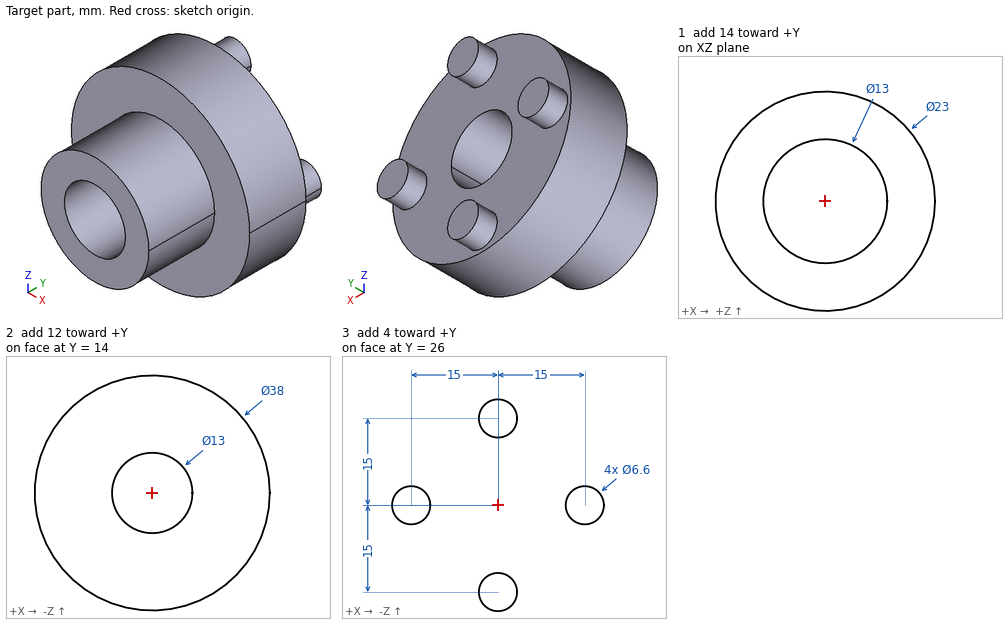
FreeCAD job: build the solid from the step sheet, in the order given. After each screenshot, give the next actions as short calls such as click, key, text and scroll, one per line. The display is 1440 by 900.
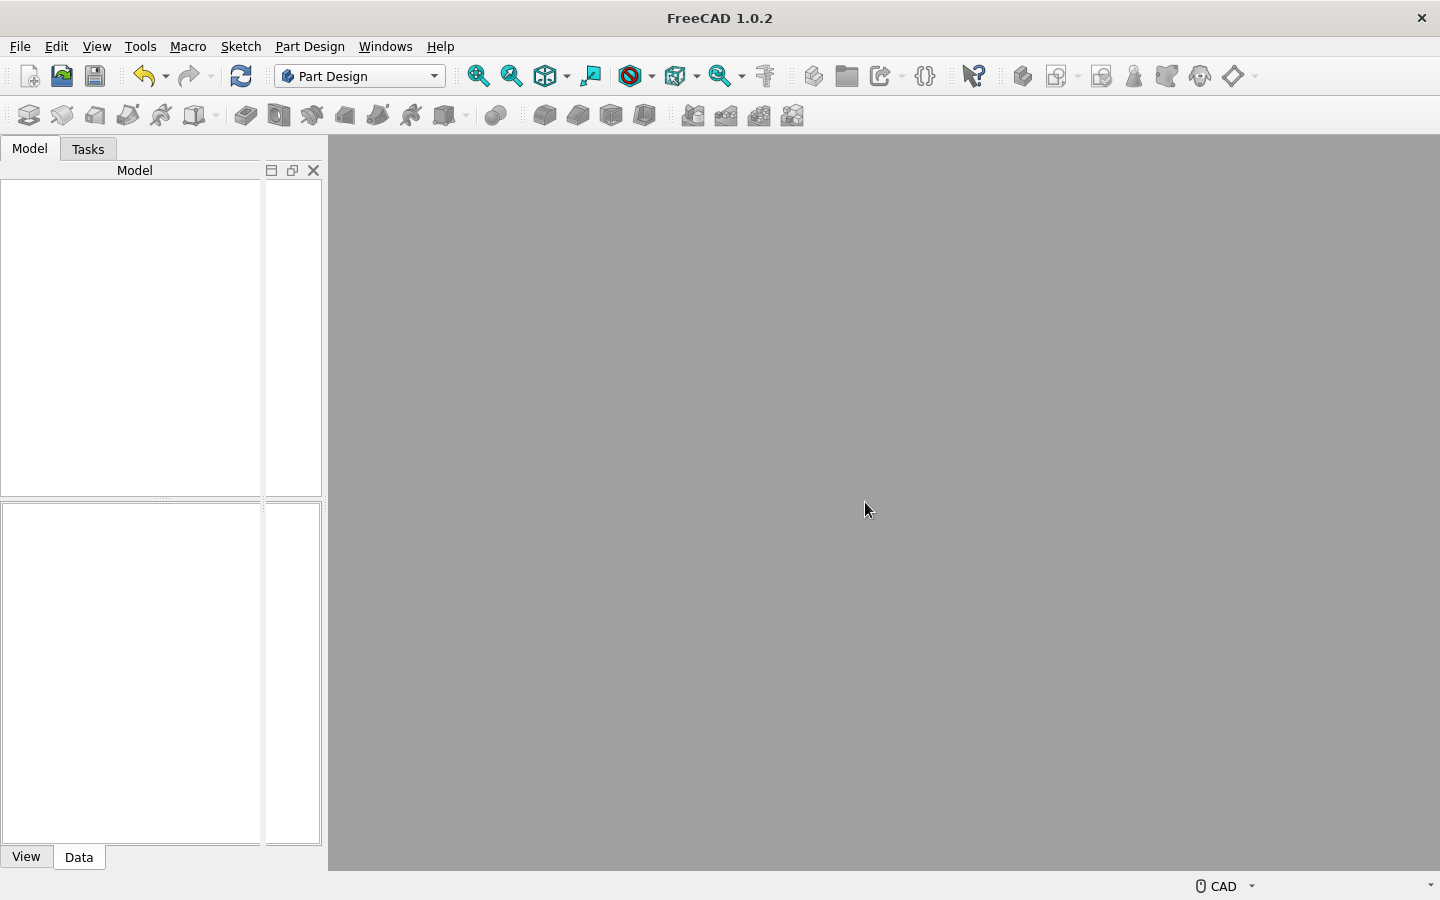
click(29, 76)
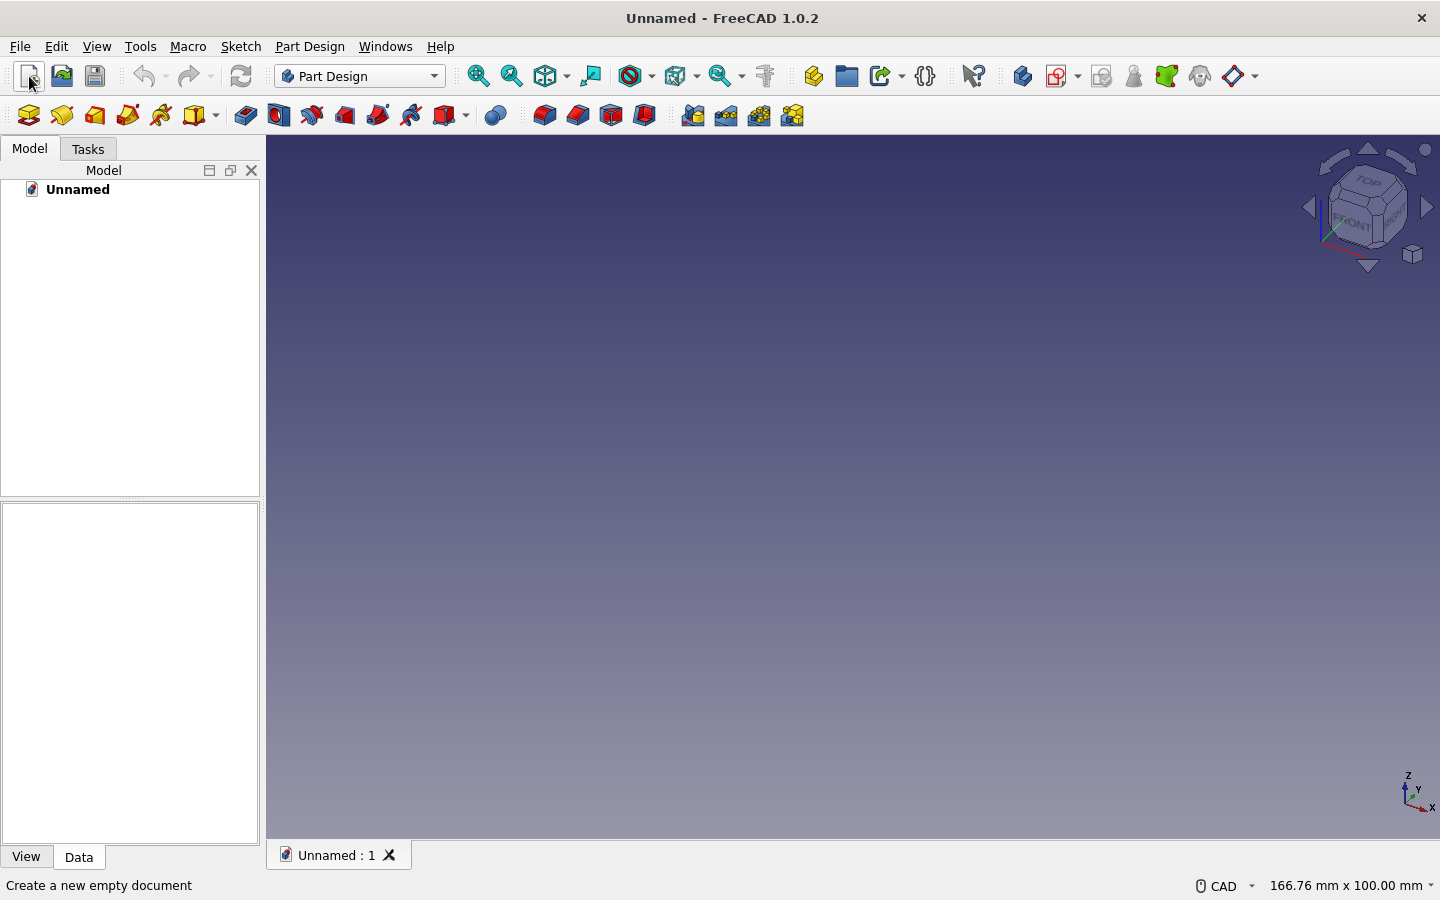
click(1056, 76)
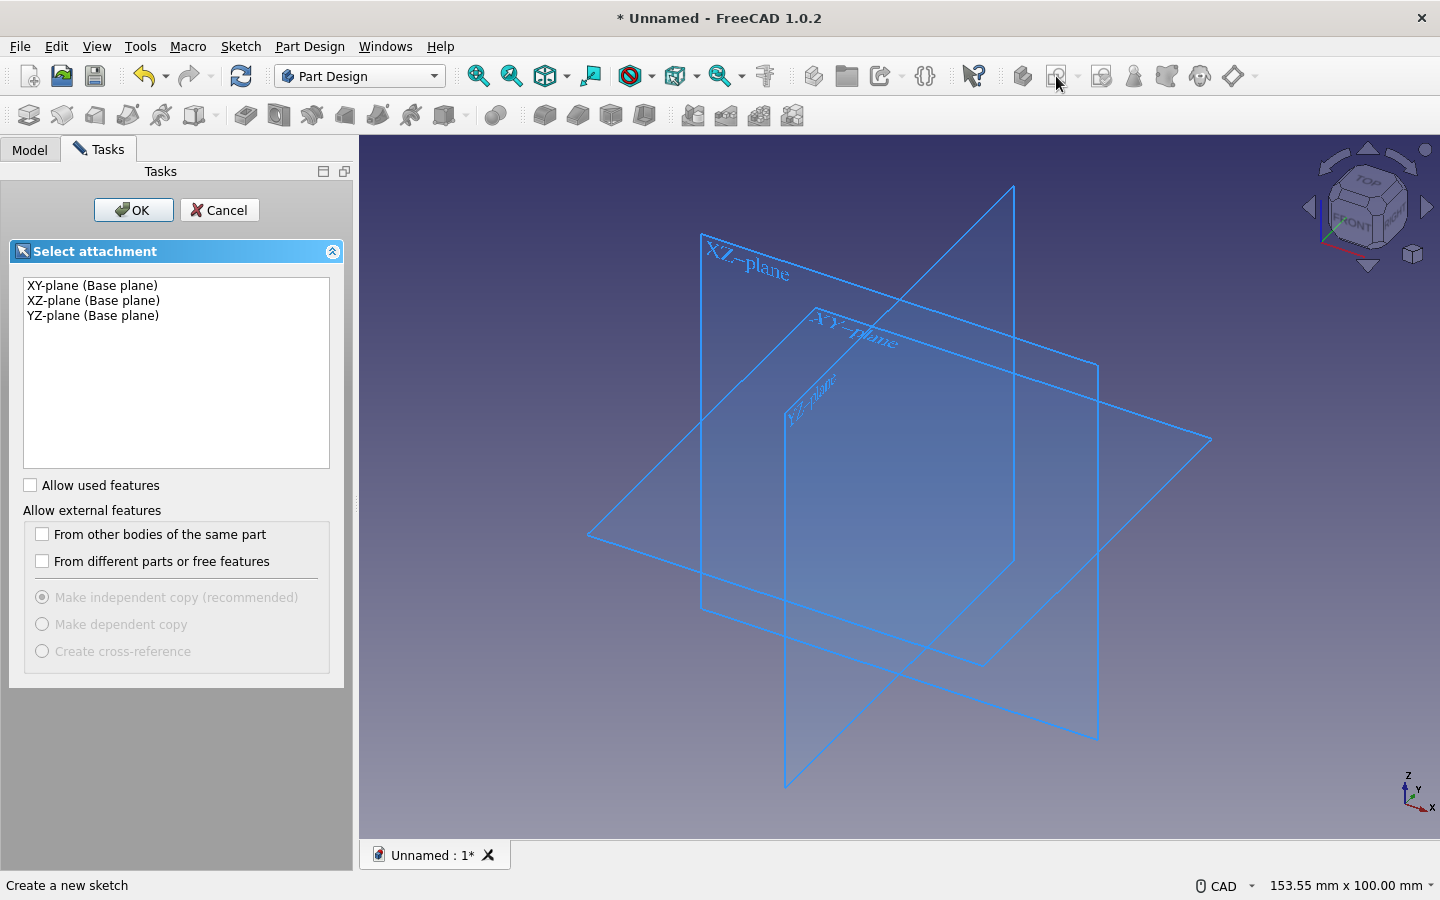
click(84, 300)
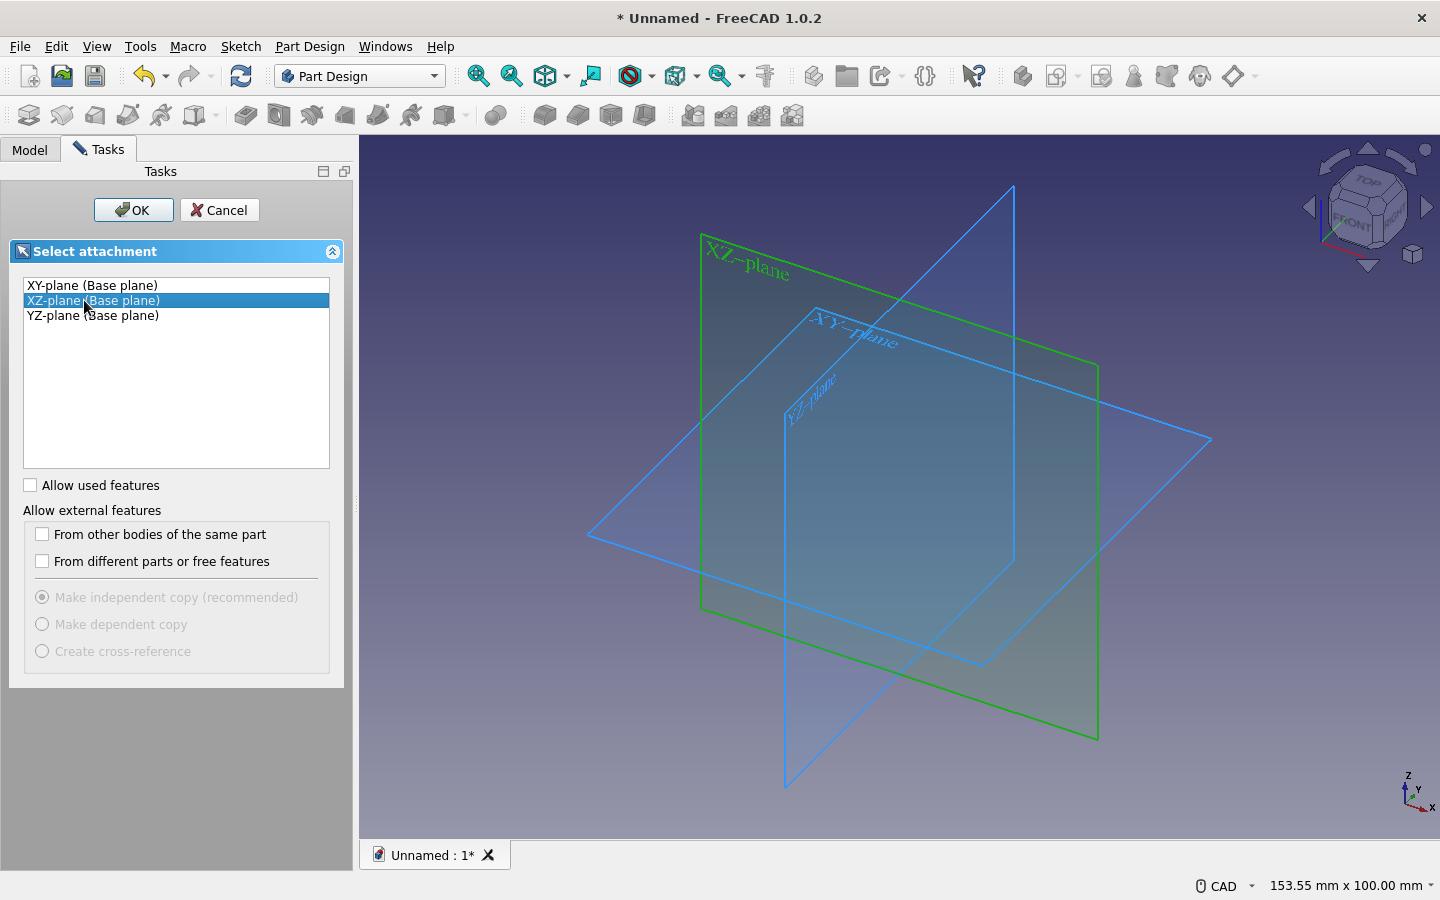
click(134, 210)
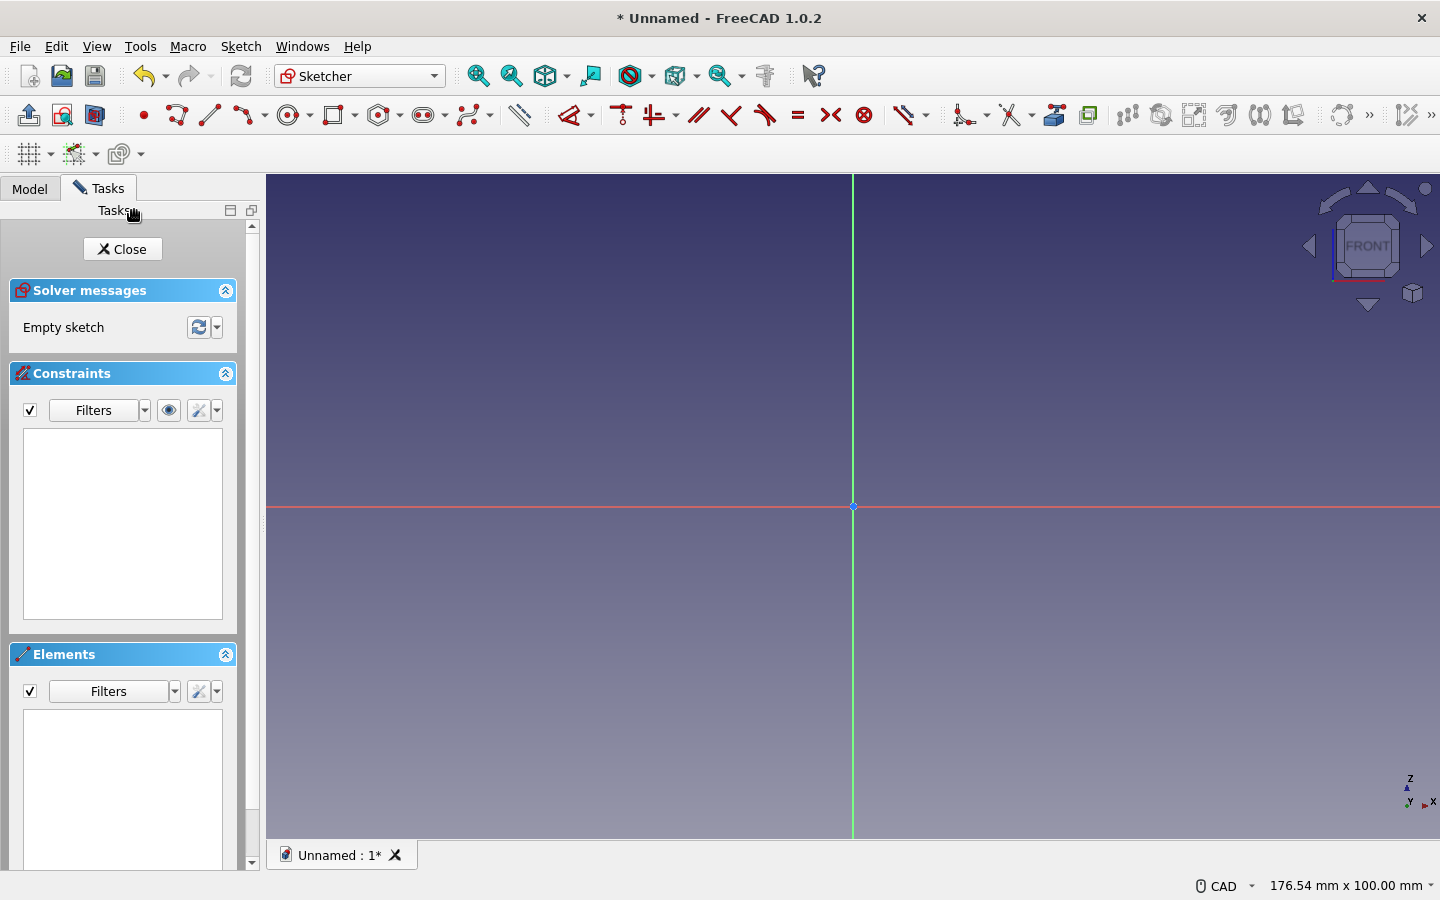
scroll(893, 507, up, 5)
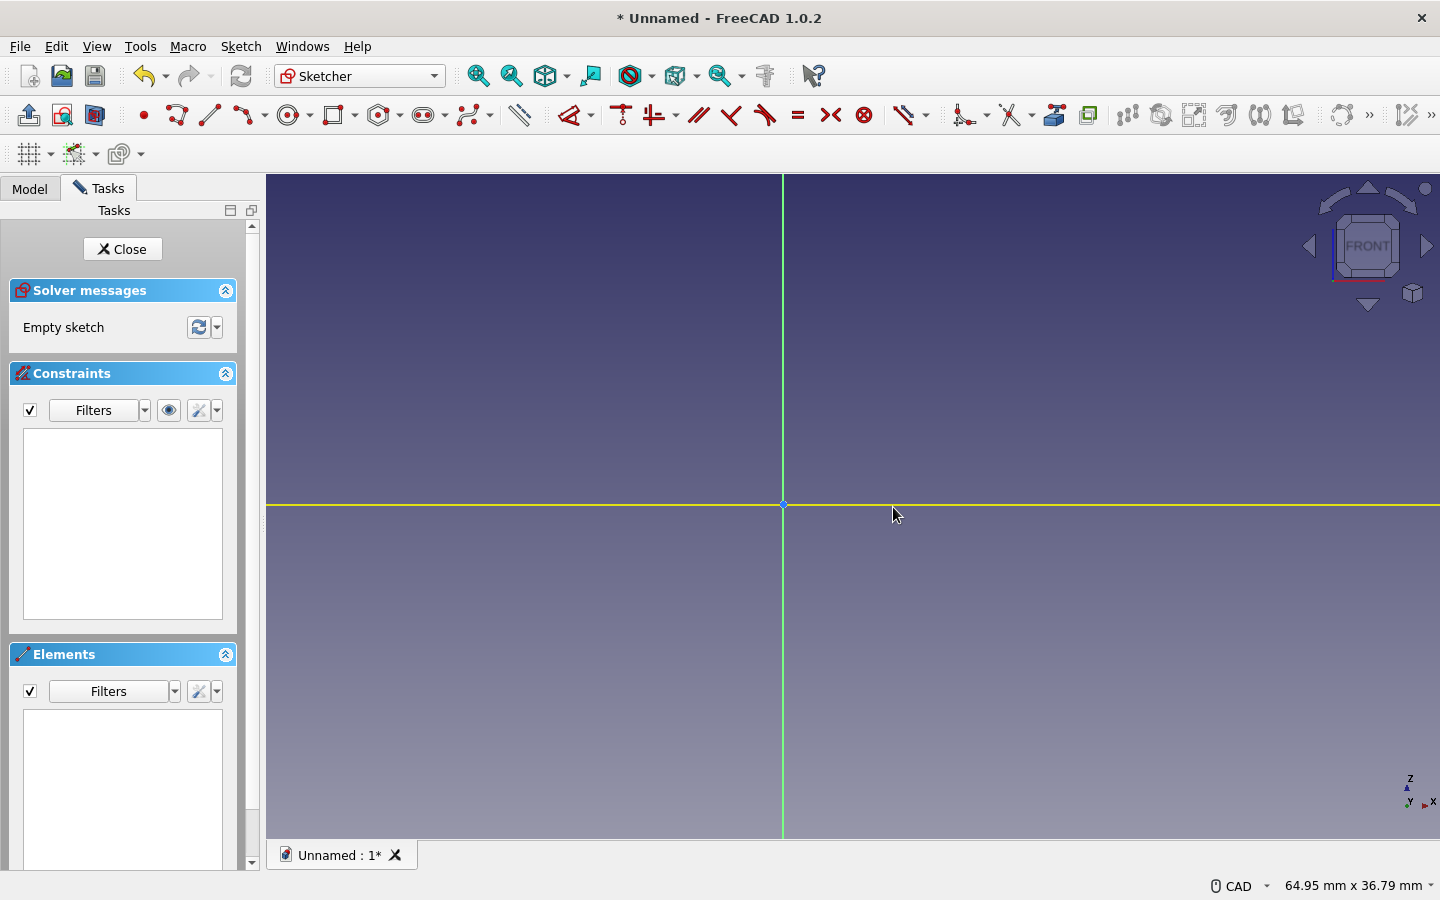
click(288, 116)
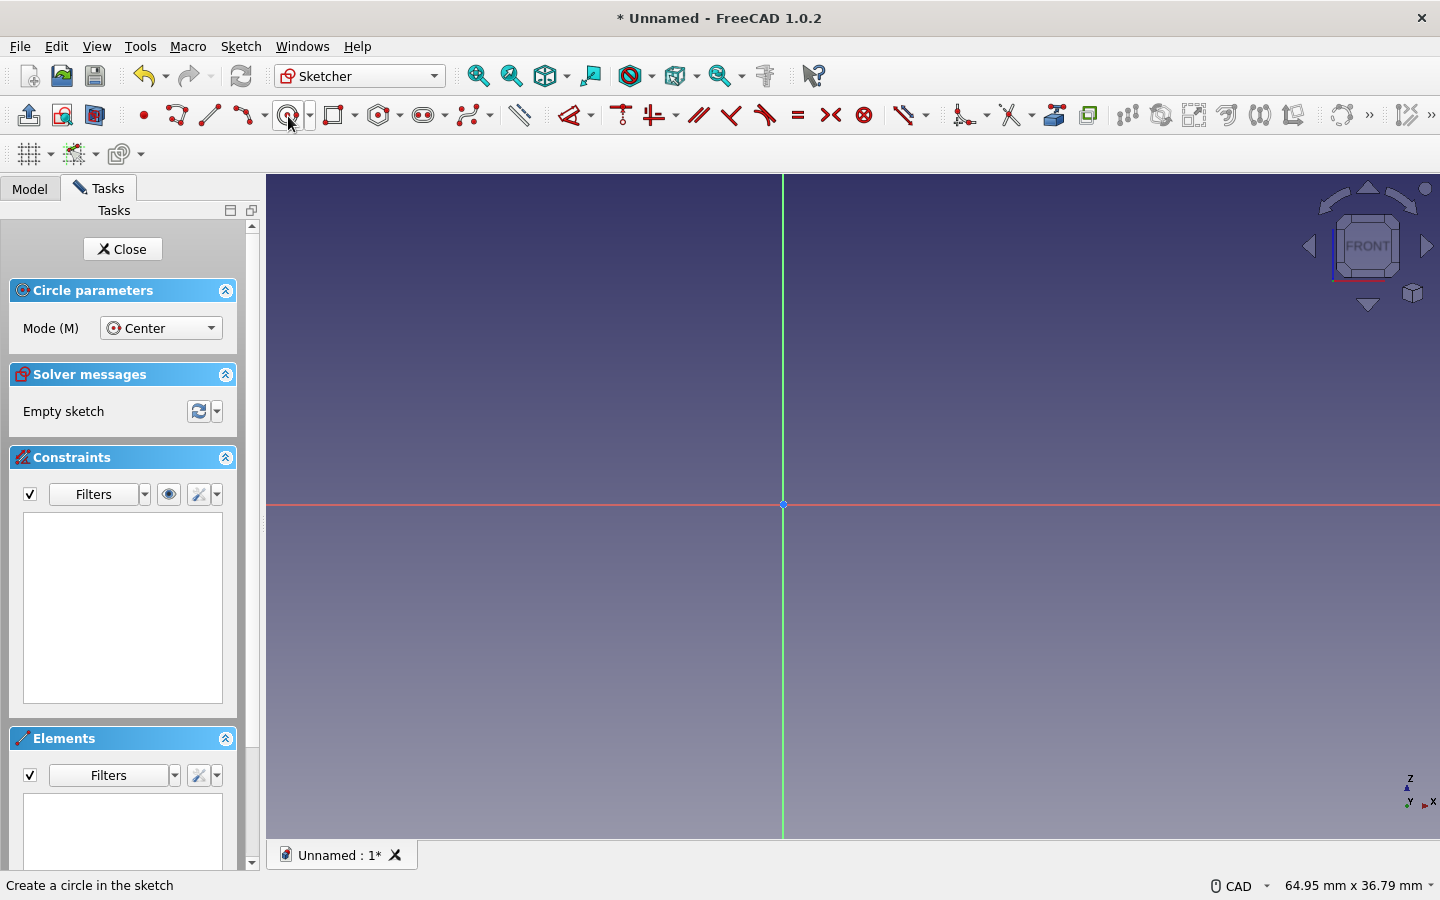
click(783, 505)
click(930, 358)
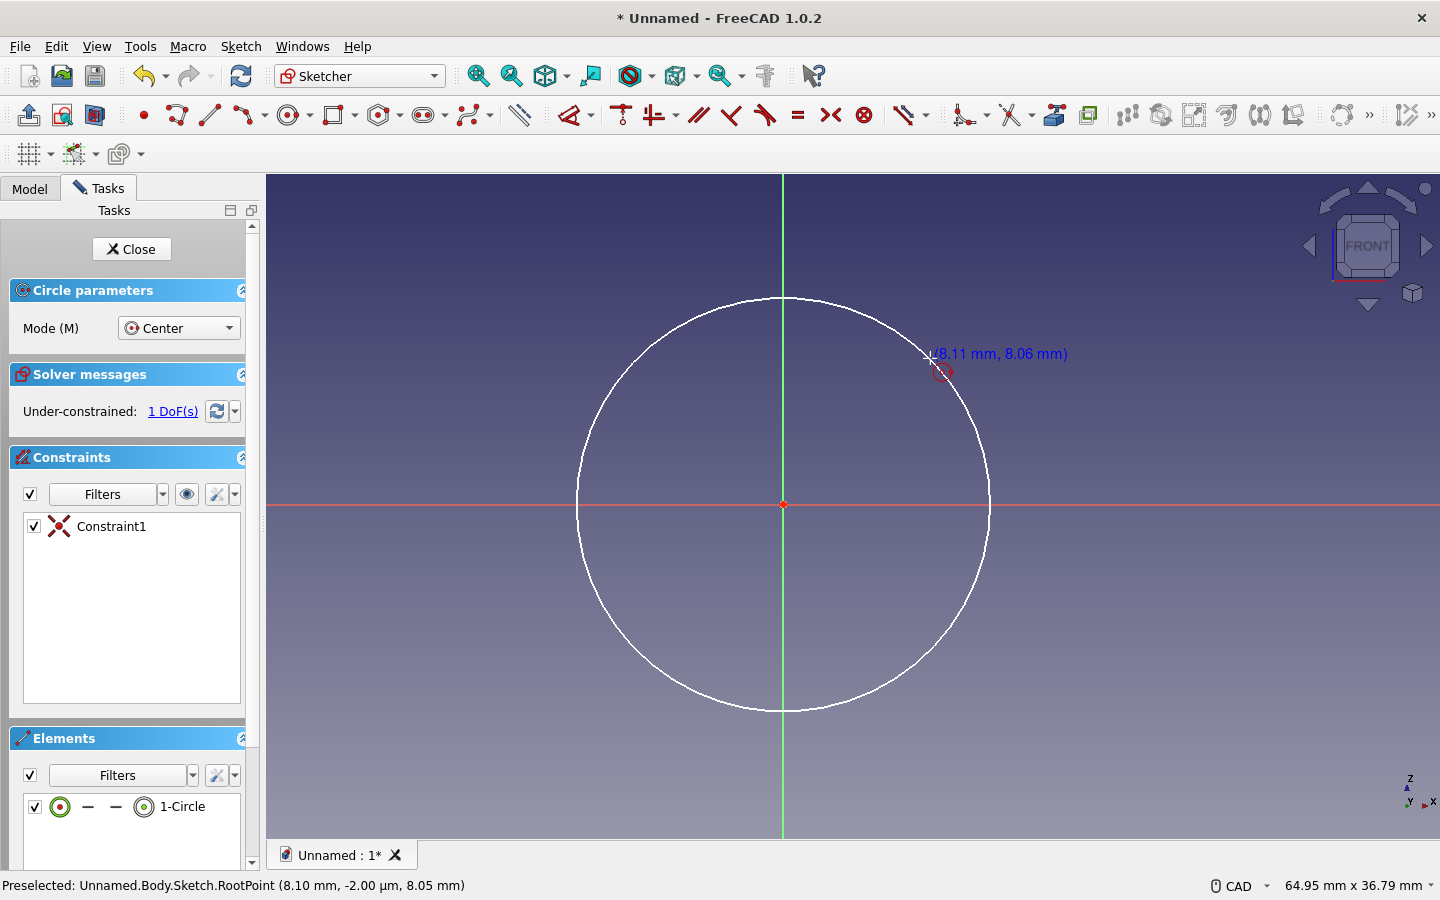
click(783, 505)
click(866, 422)
key(Escape)